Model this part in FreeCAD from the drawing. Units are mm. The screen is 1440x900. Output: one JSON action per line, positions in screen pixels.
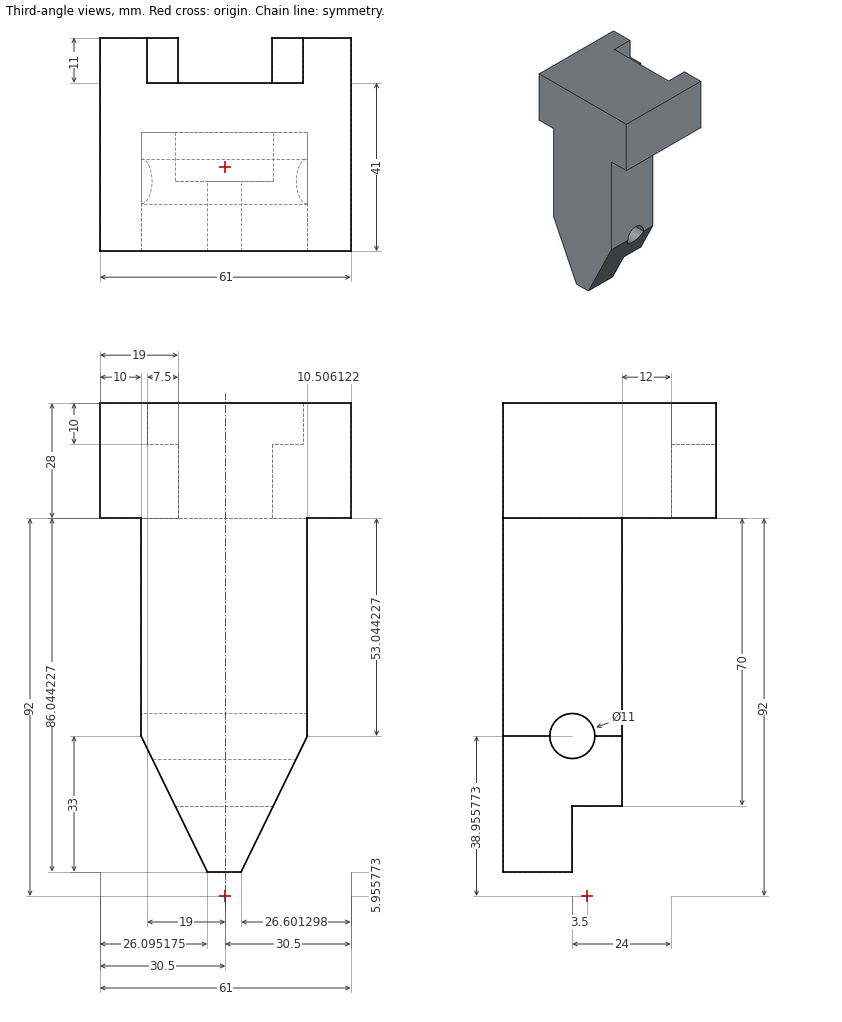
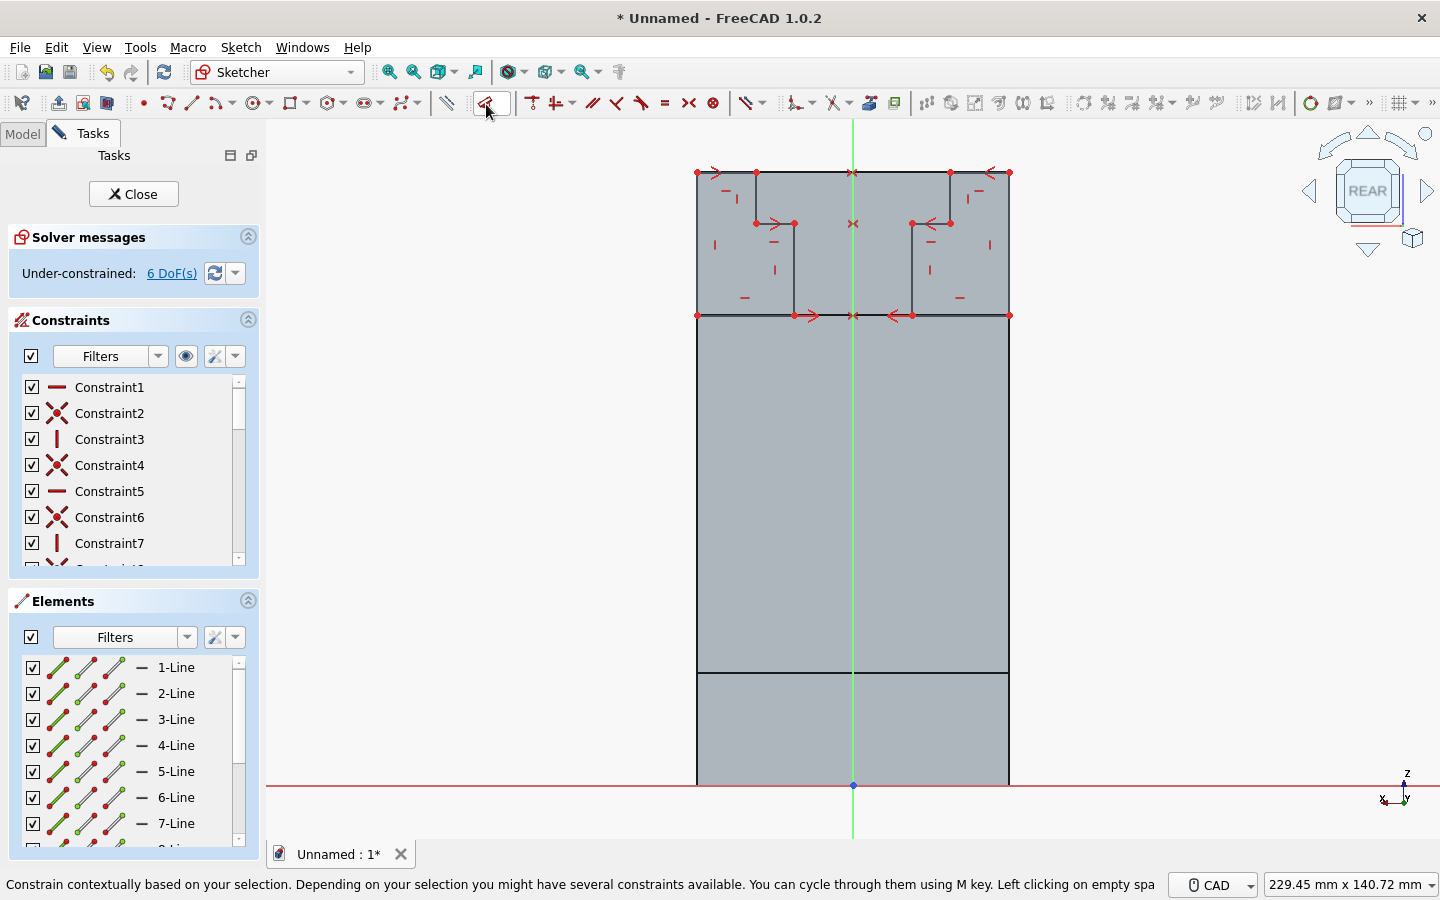
{"action": "left_click", "coordinate": [941, 316]}
{"action": "left_click", "coordinate": [960, 282]}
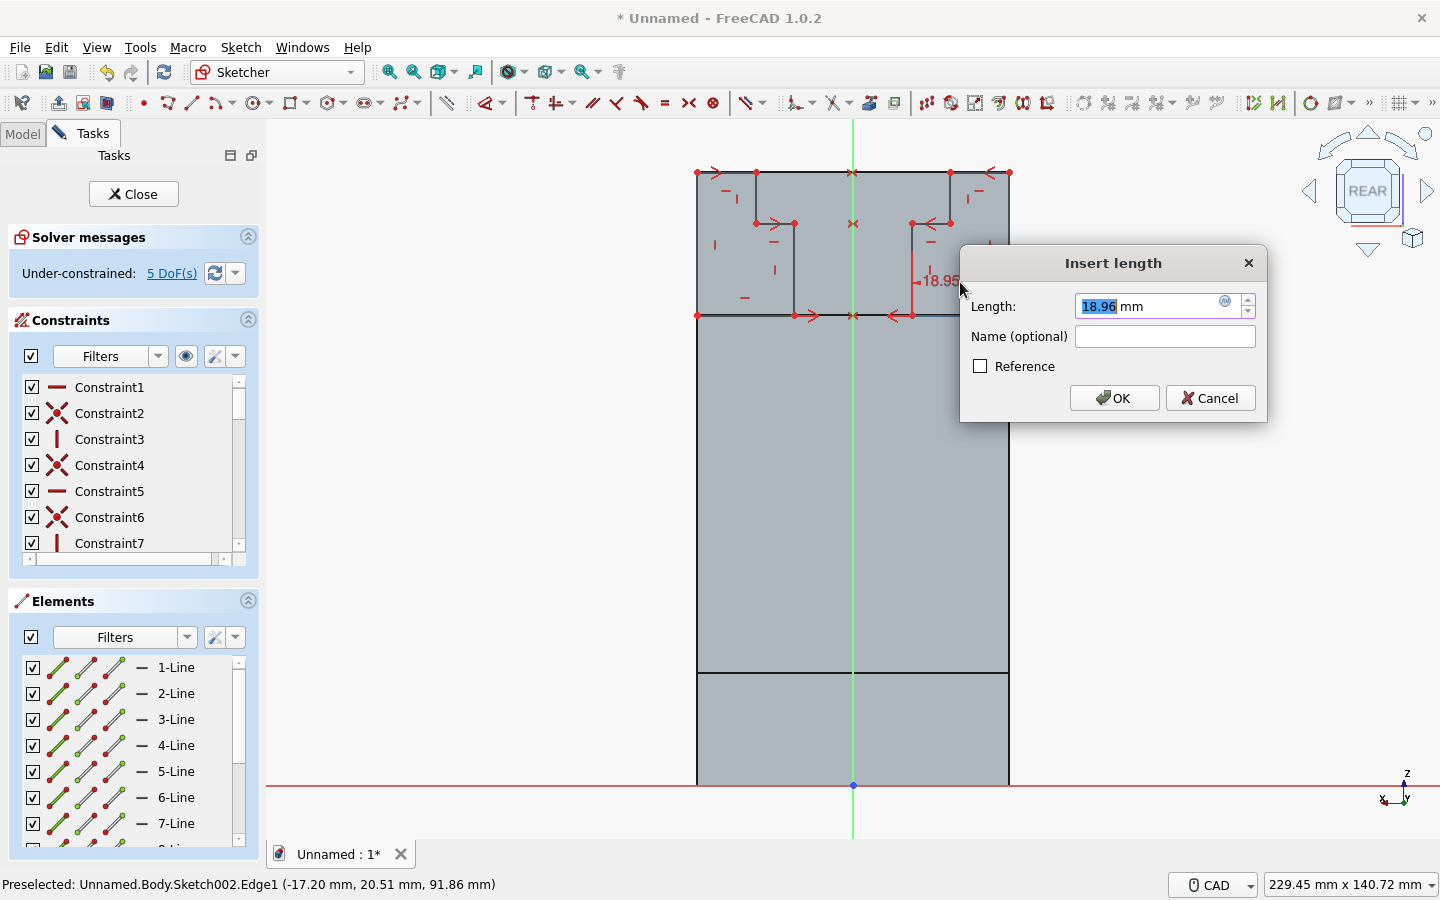
{"action": "type", "text": "19"}
{"action": "key", "text": "Return"}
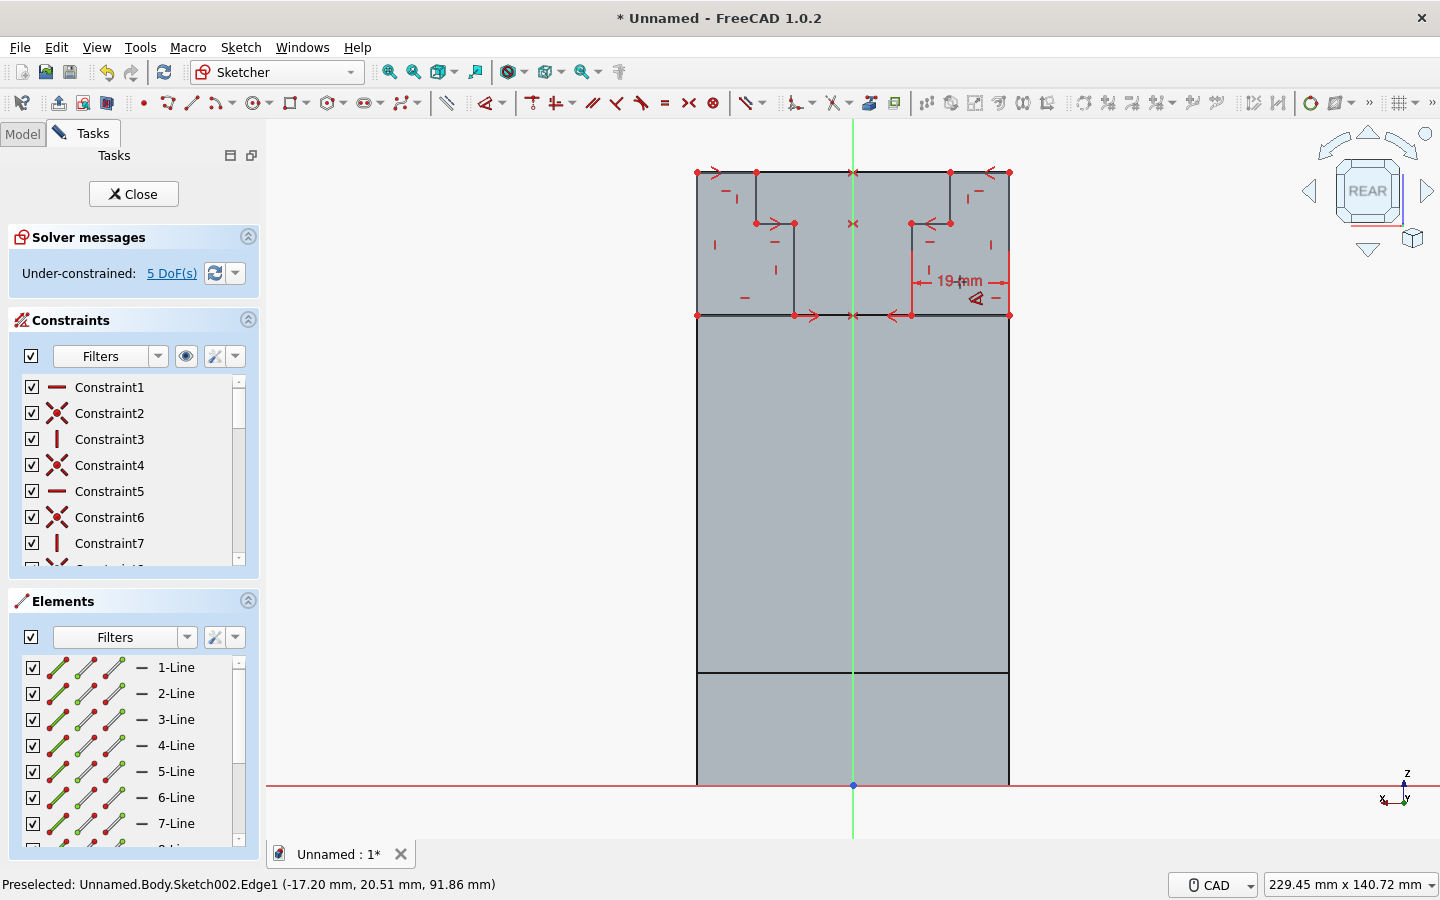
{"action": "left_click", "coordinate": [1009, 273]}
{"action": "left_click", "coordinate": [1043, 245]}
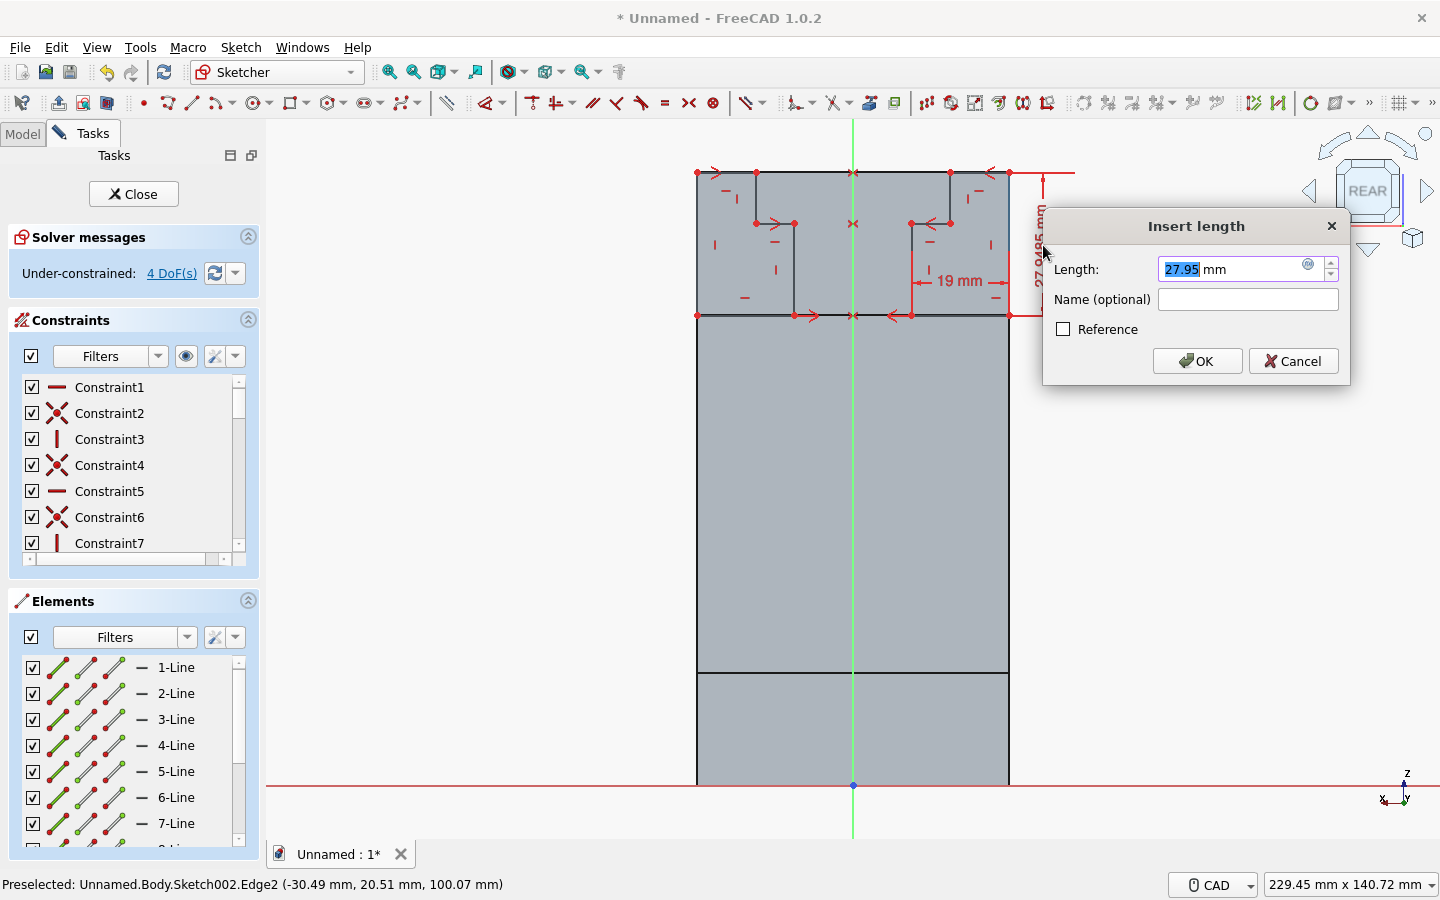
{"action": "type", "text": "28"}
{"action": "key", "text": "Return"}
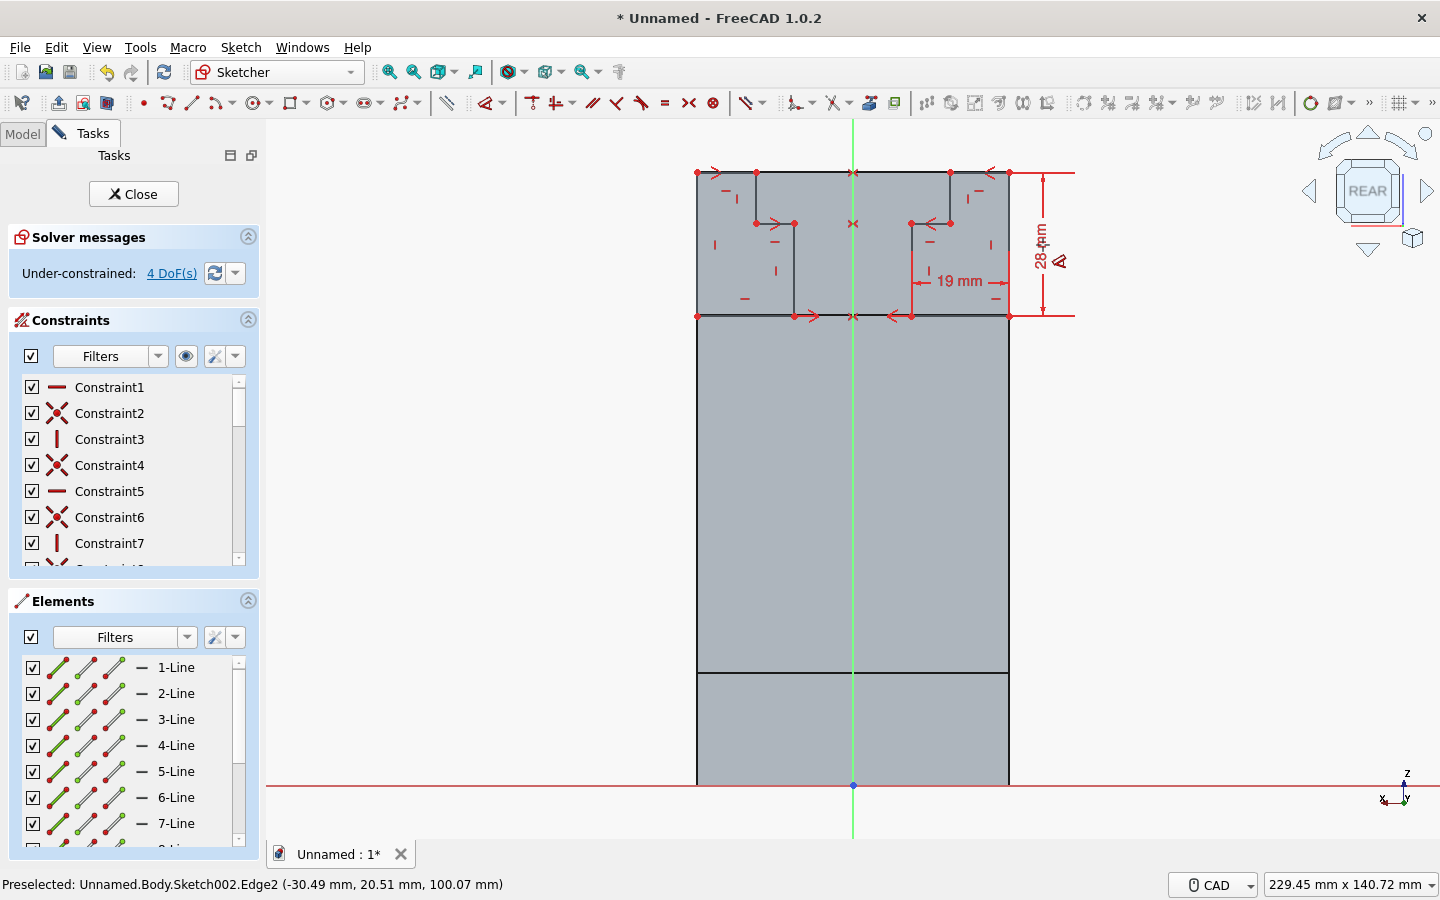
{"action": "left_click", "coordinate": [950, 188]}
{"action": "left_click", "coordinate": [984, 198]}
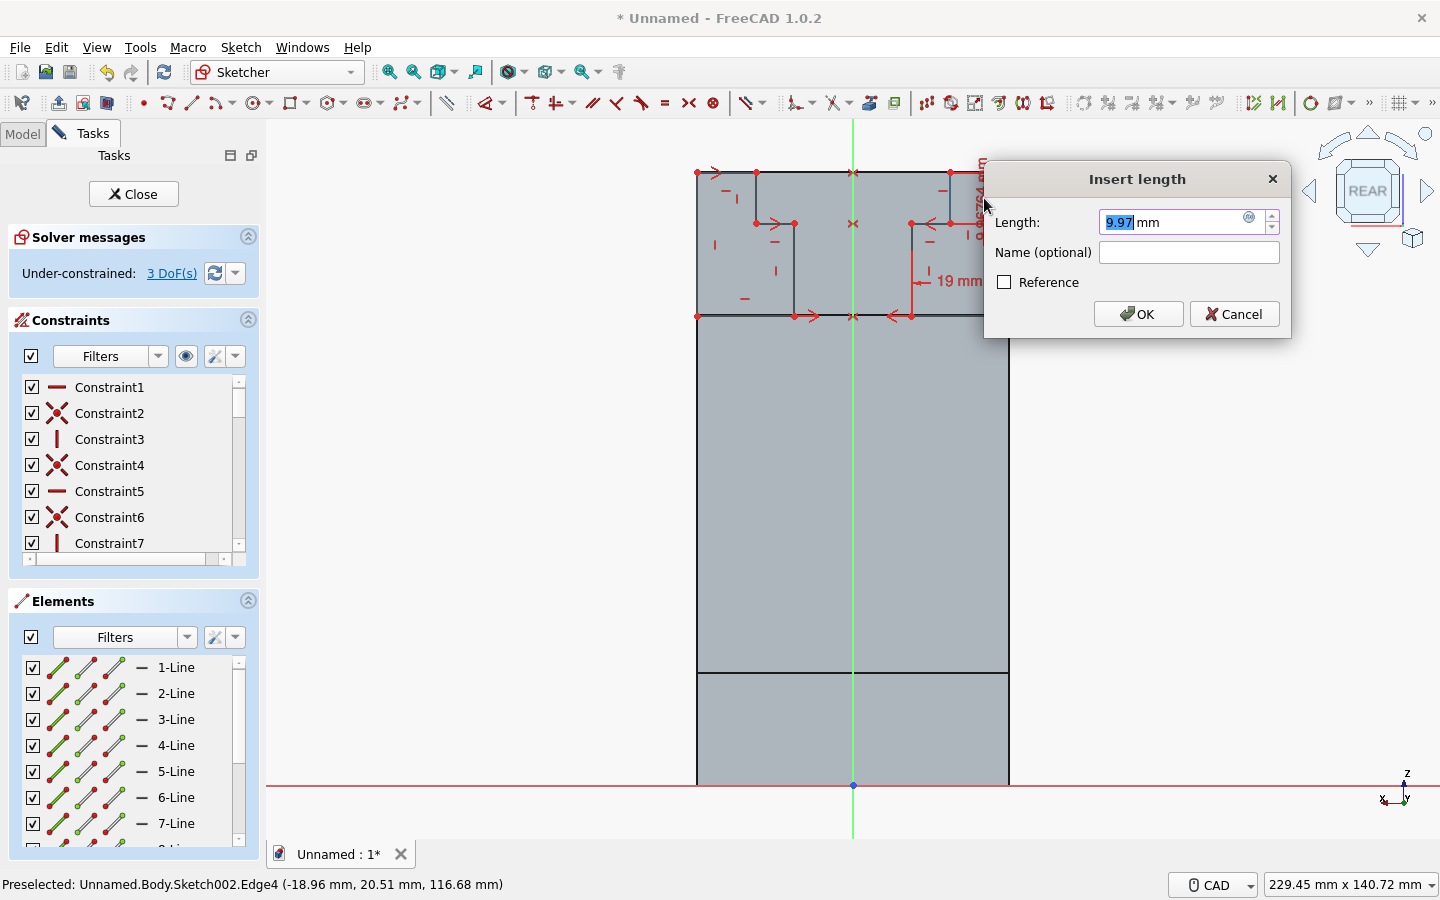
{"action": "type", "text": "10"}
{"action": "key", "text": "Return"}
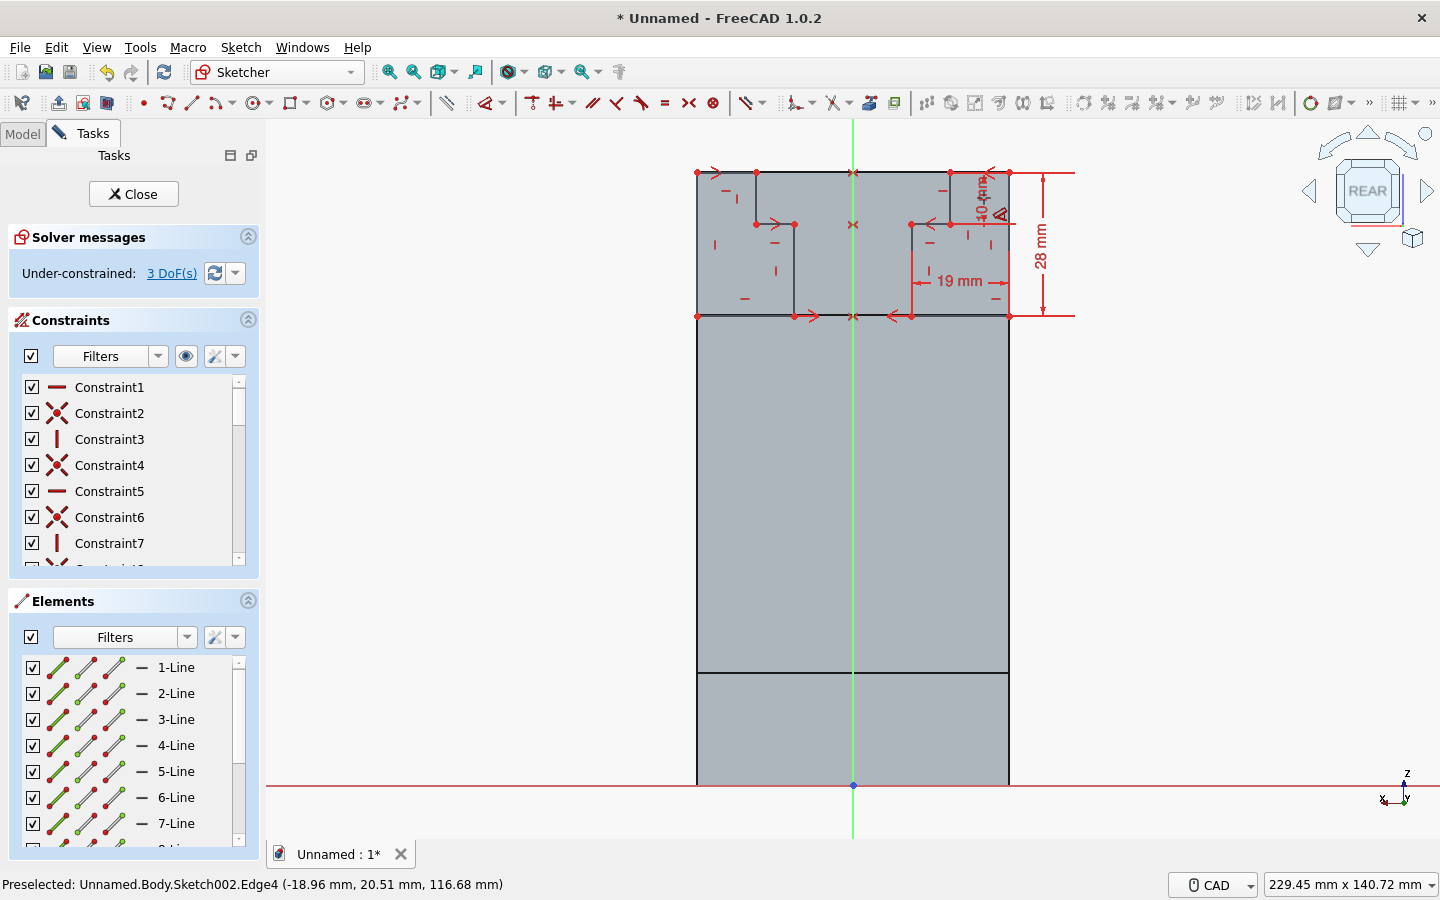
{"action": "left_click", "coordinate": [939, 224]}
{"action": "left_click", "coordinate": [931, 258]}